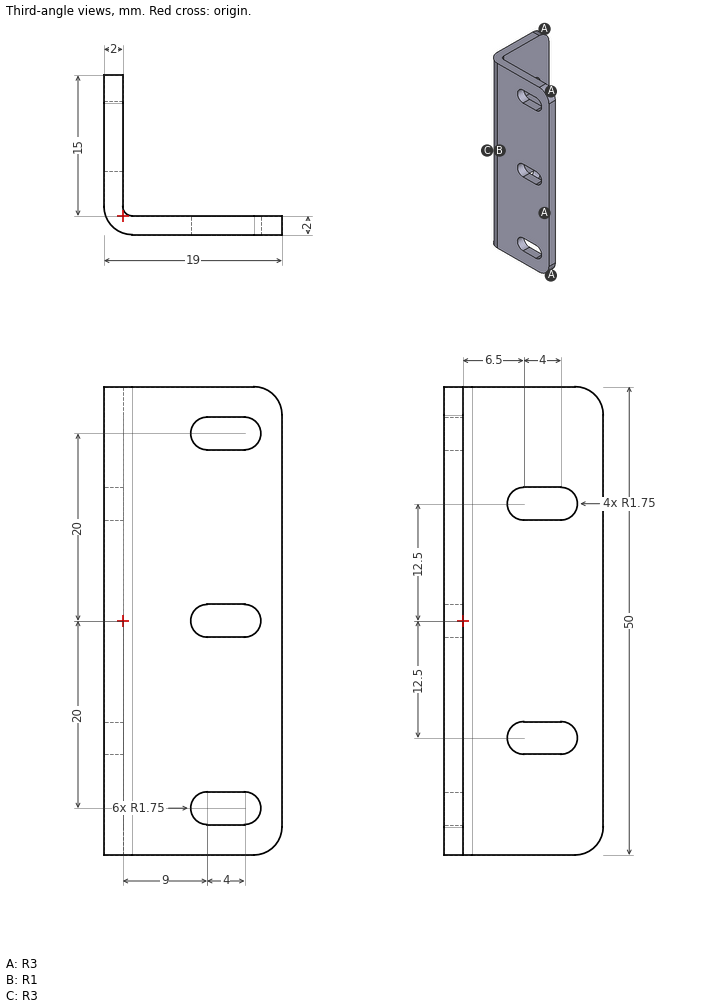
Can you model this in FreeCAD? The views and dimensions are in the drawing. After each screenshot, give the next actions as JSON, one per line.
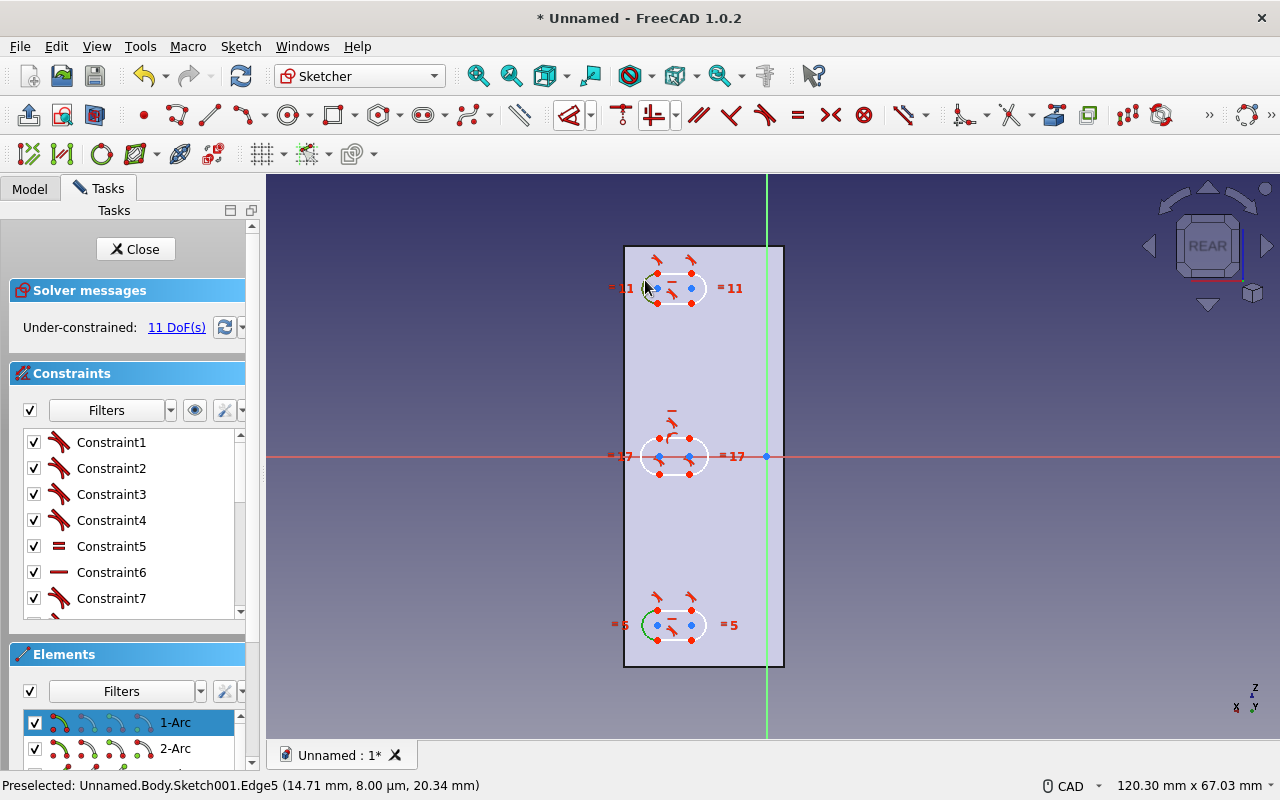
{"action": "scroll", "coordinate": [644, 446], "scroll_direction": "up", "scroll_amount": 2}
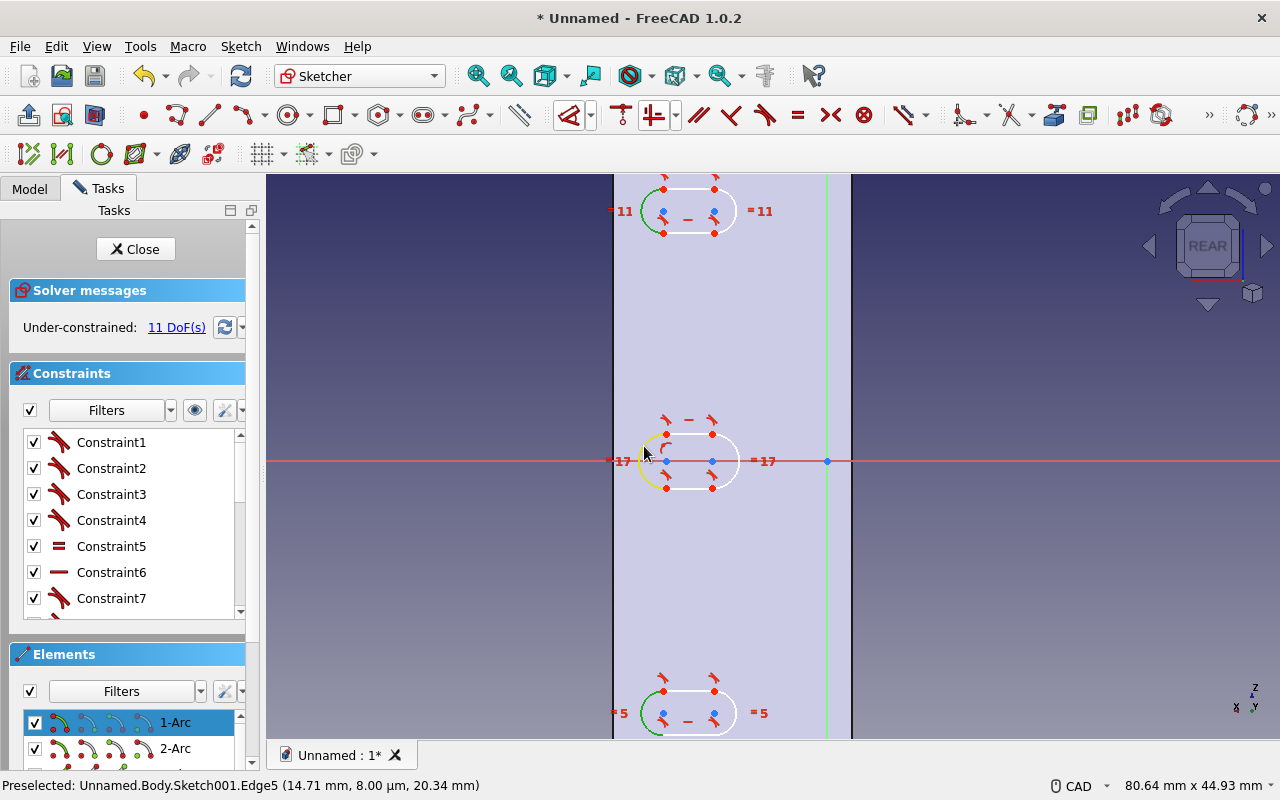
{"action": "left_click", "coordinate": [644, 445]}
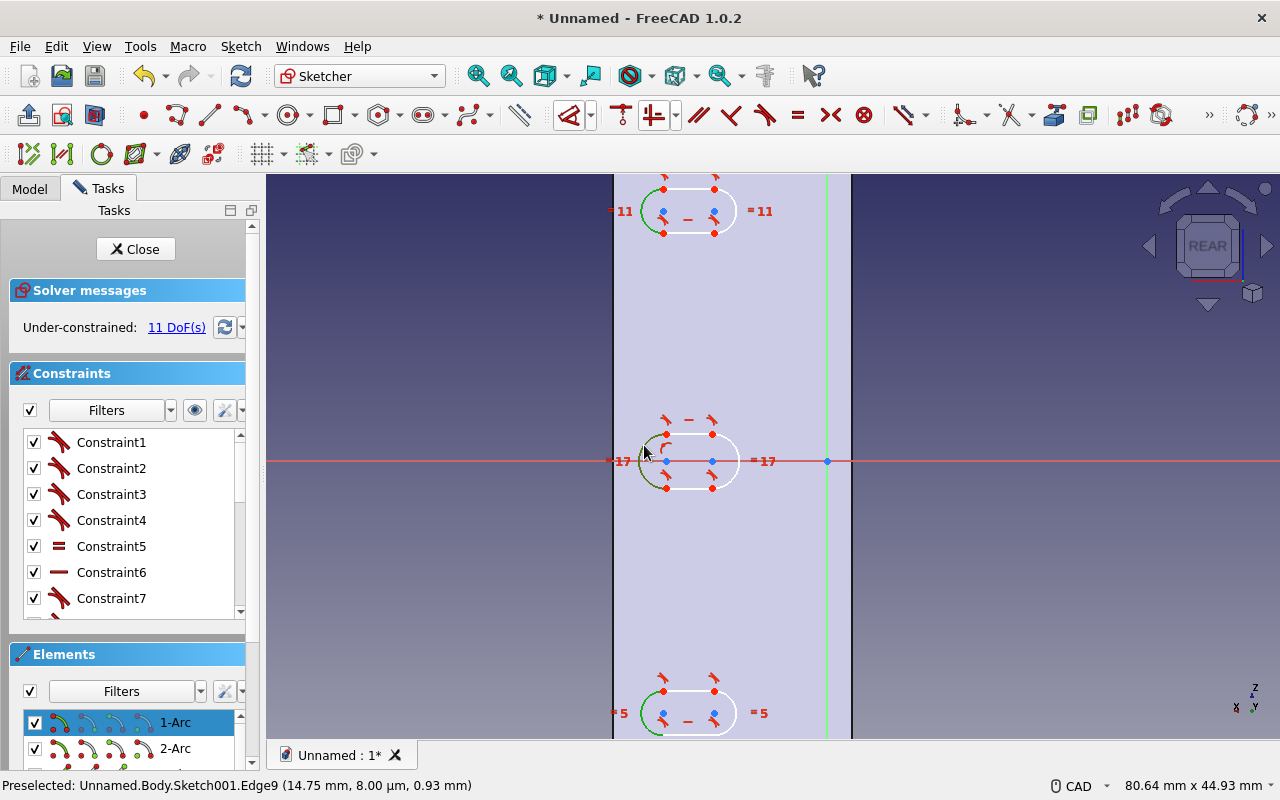
{"action": "left_click", "coordinate": [798, 116]}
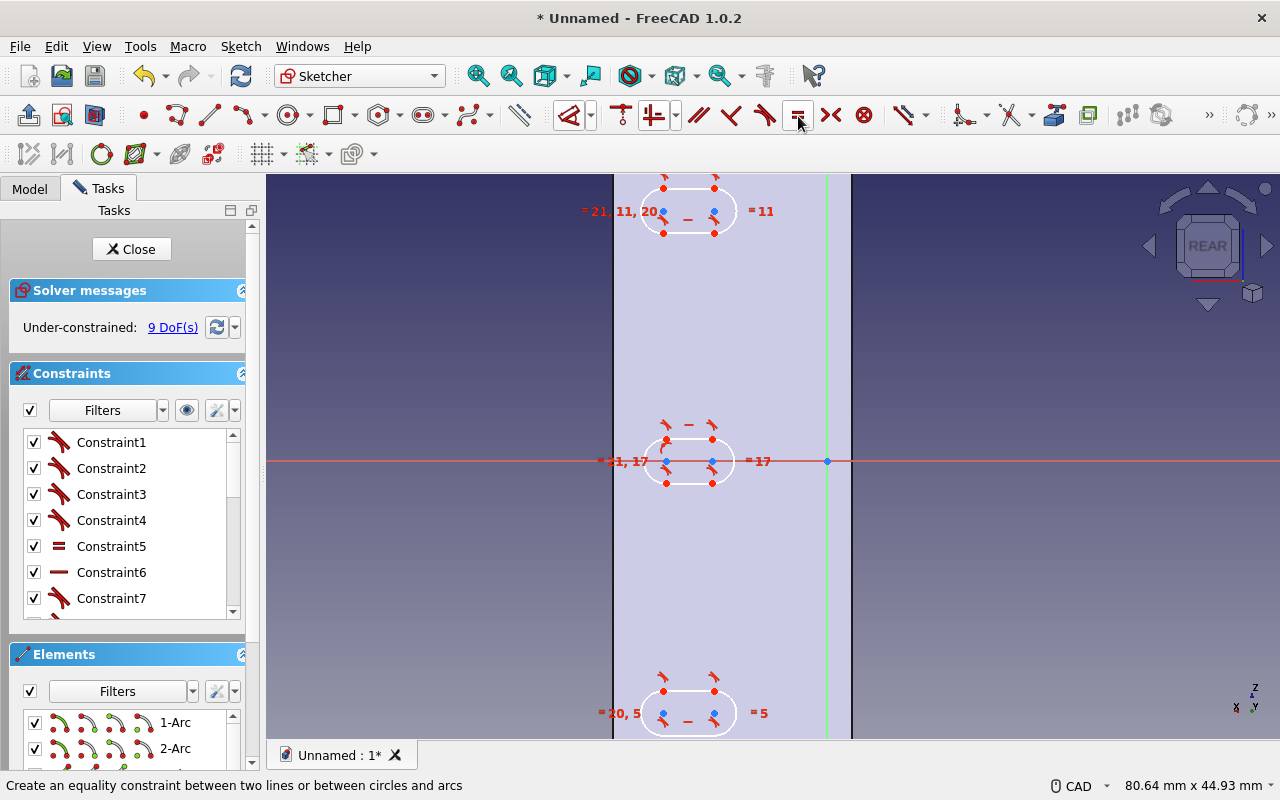
{"action": "scroll", "coordinate": [645, 700], "scroll_direction": "up", "scroll_amount": 3}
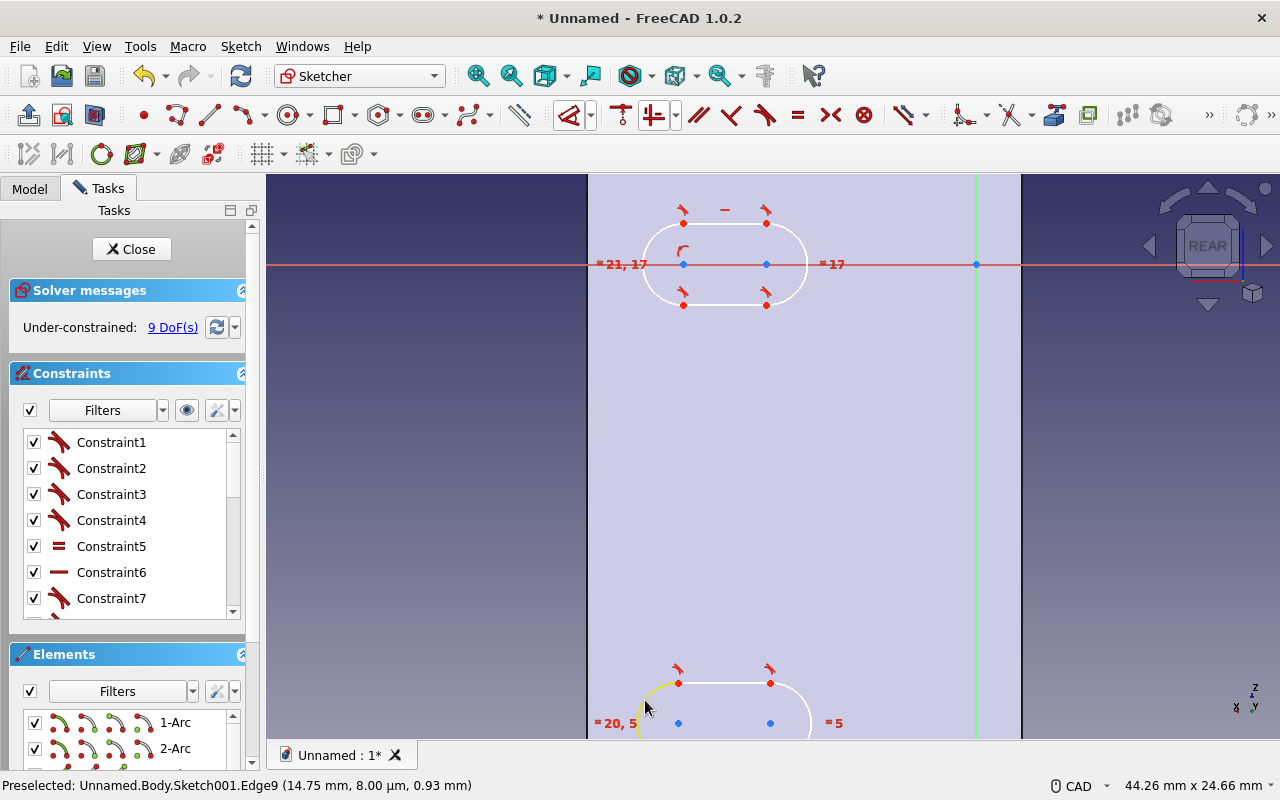
{"action": "left_click", "coordinate": [645, 700]}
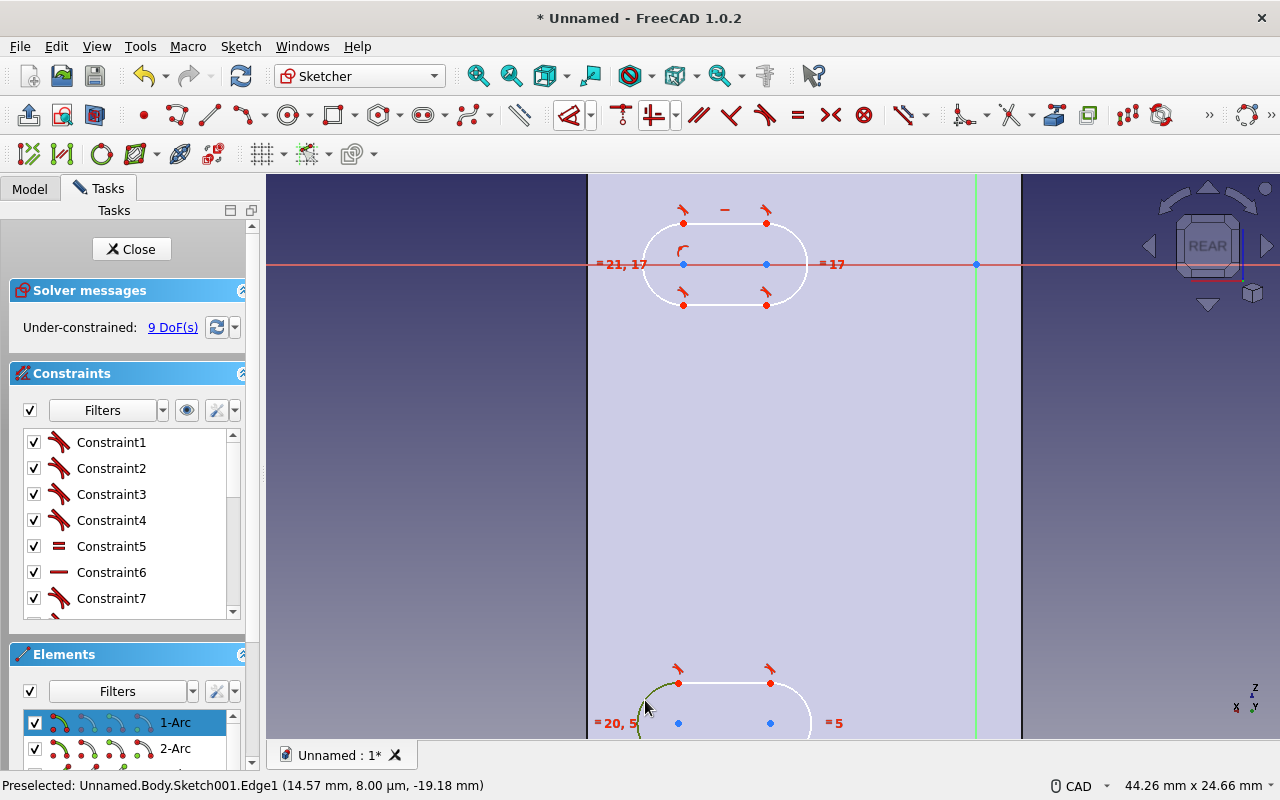
{"action": "key", "text": "k r"}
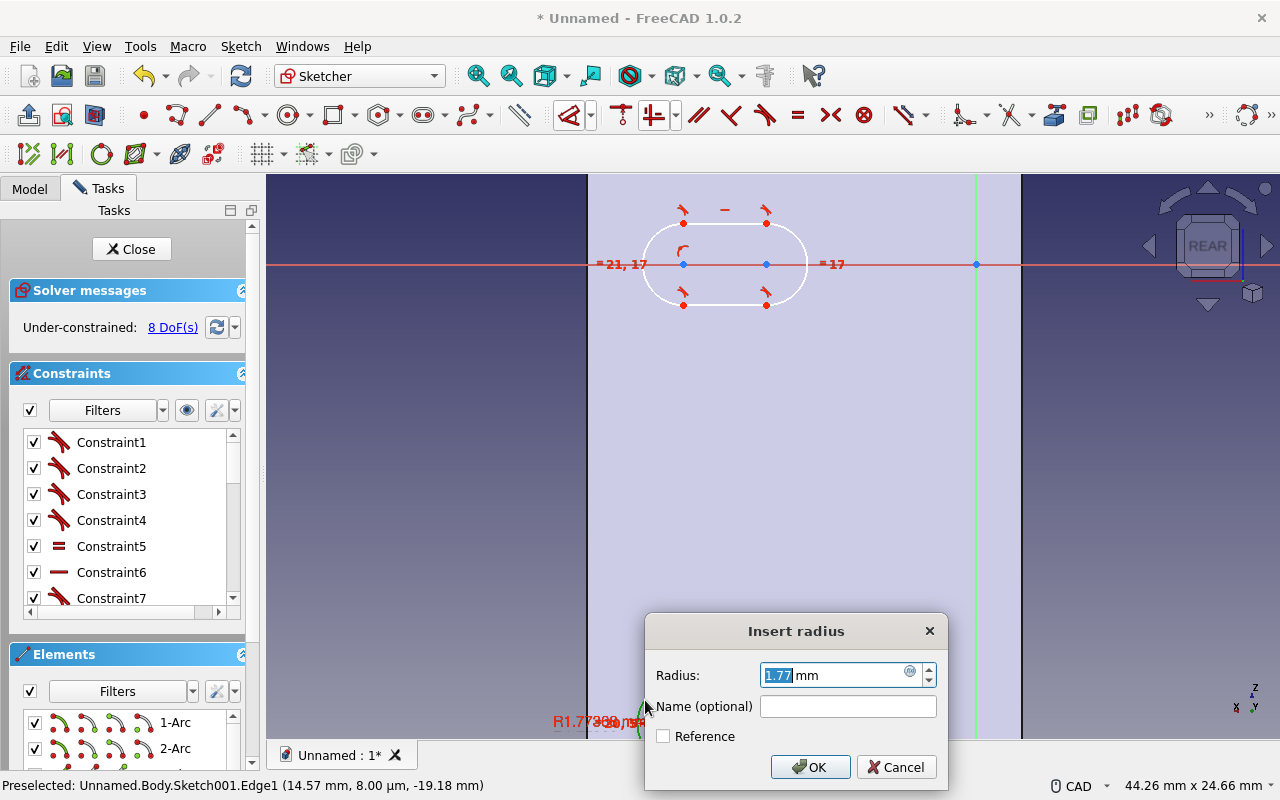
{"action": "type", "text": "1.75"}
{"action": "key", "text": "Return"}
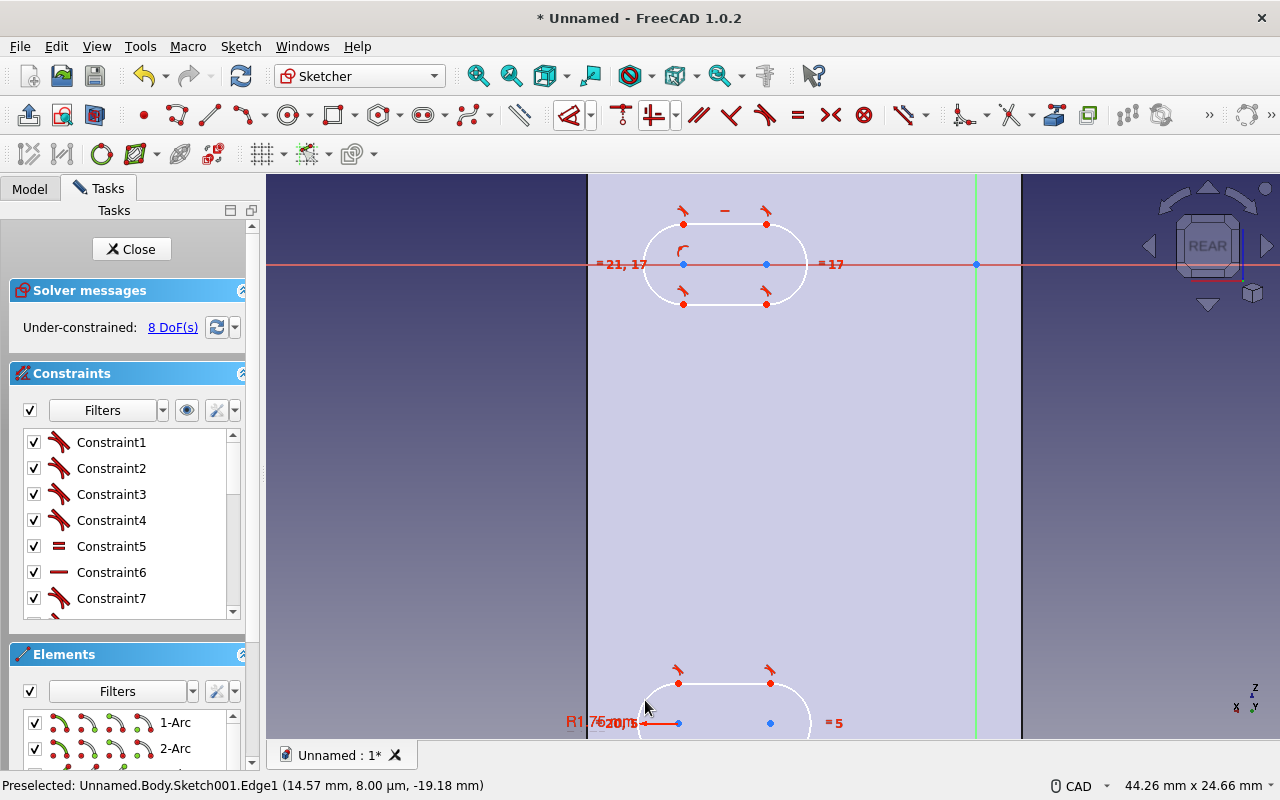
{"action": "left_click", "coordinate": [706, 684]}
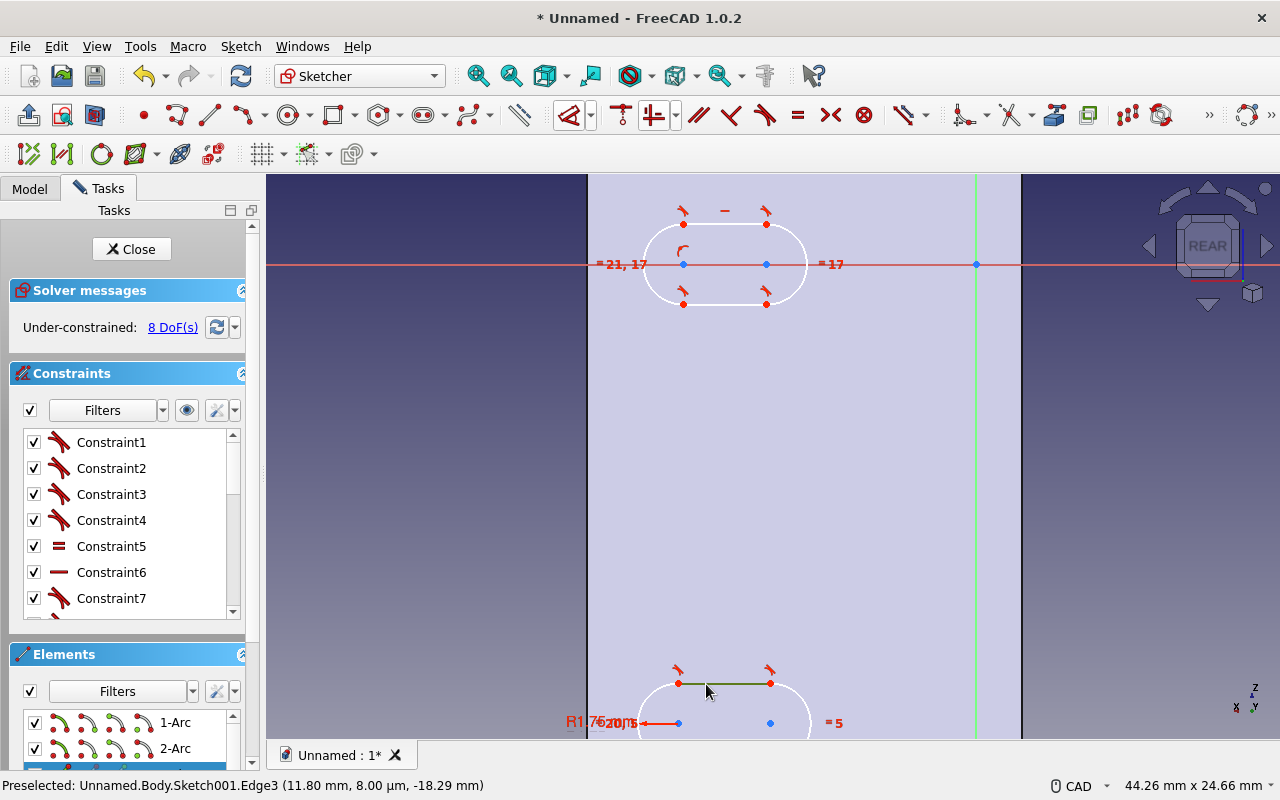
{"action": "left_click", "coordinate": [590, 116]}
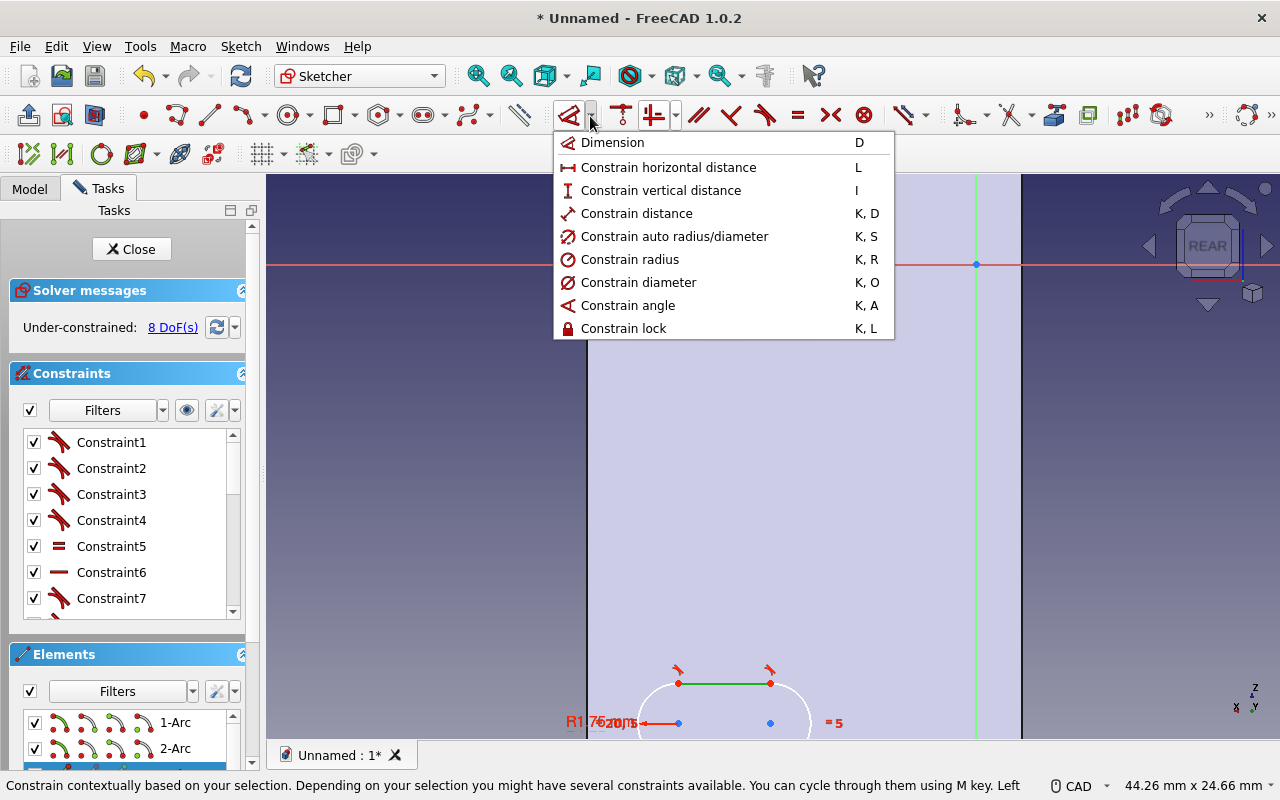
{"action": "left_click", "coordinate": [724, 168]}